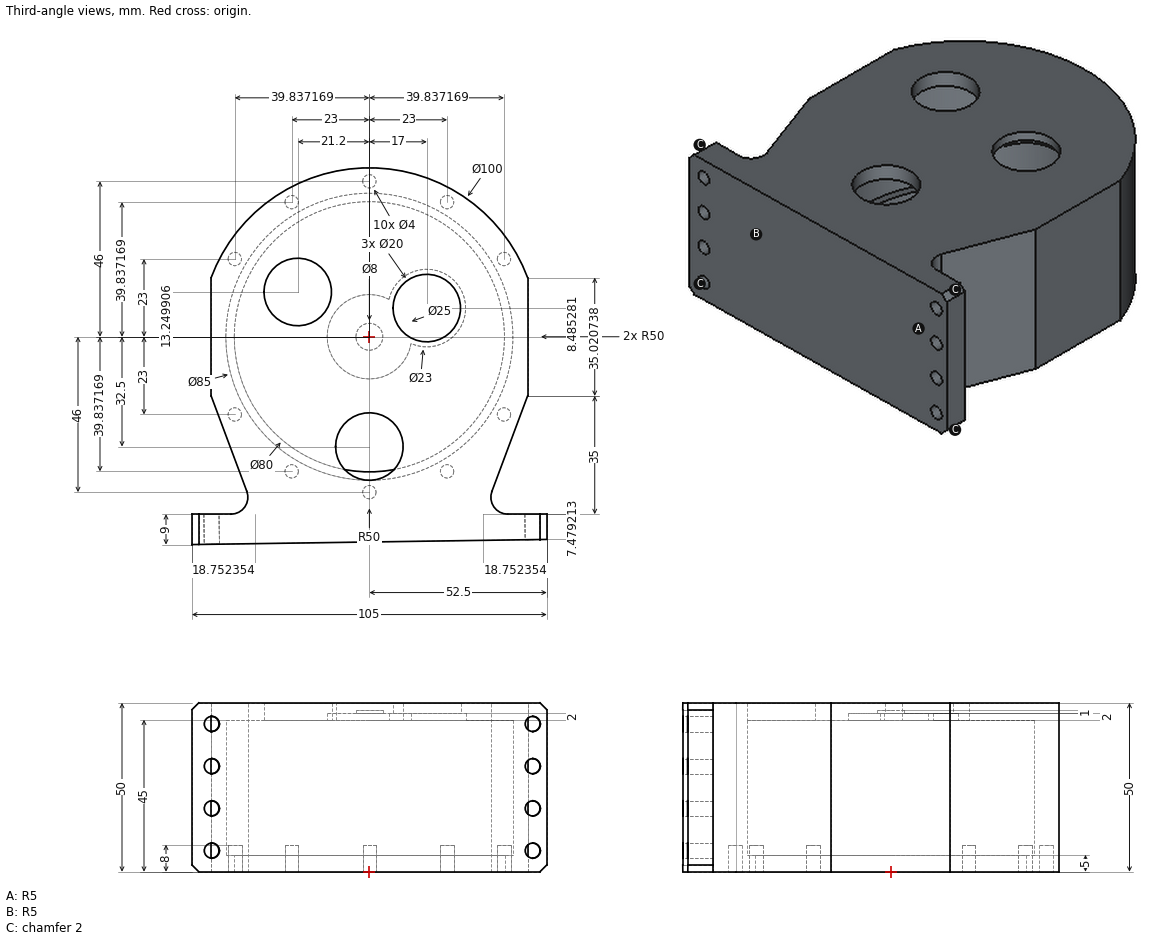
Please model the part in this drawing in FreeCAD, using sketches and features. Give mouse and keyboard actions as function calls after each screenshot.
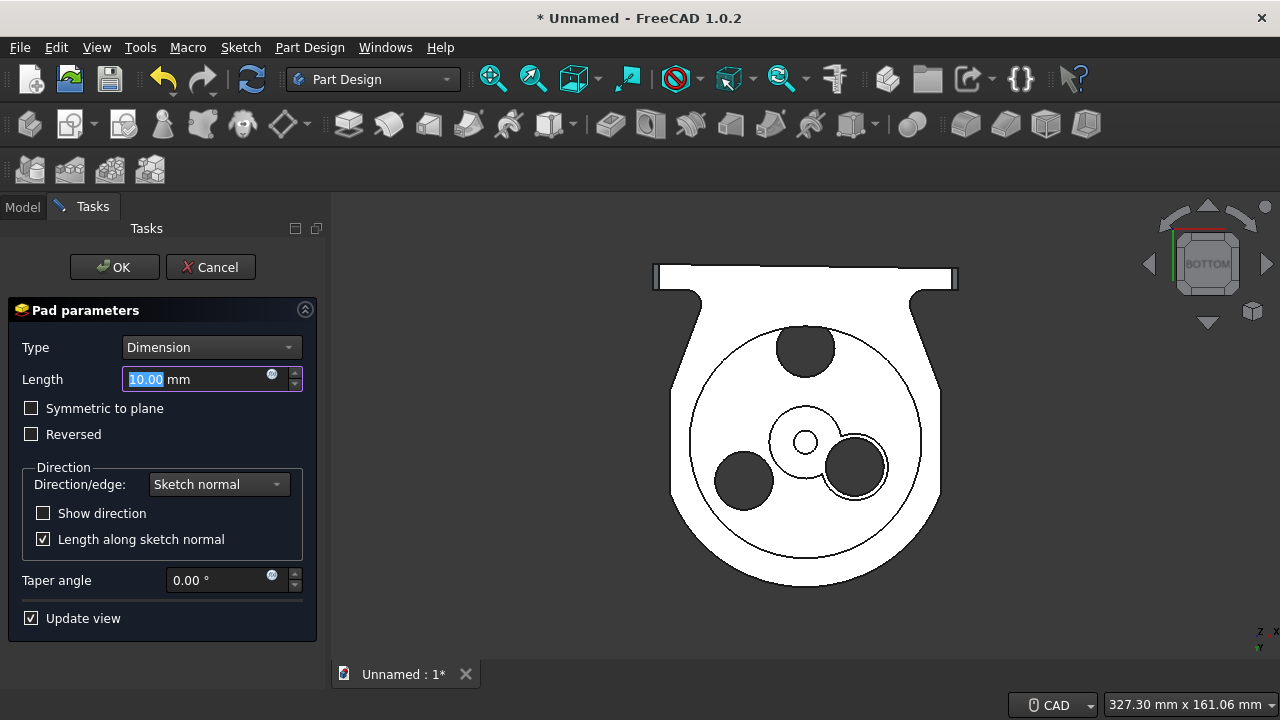
text(5)
key(Tab)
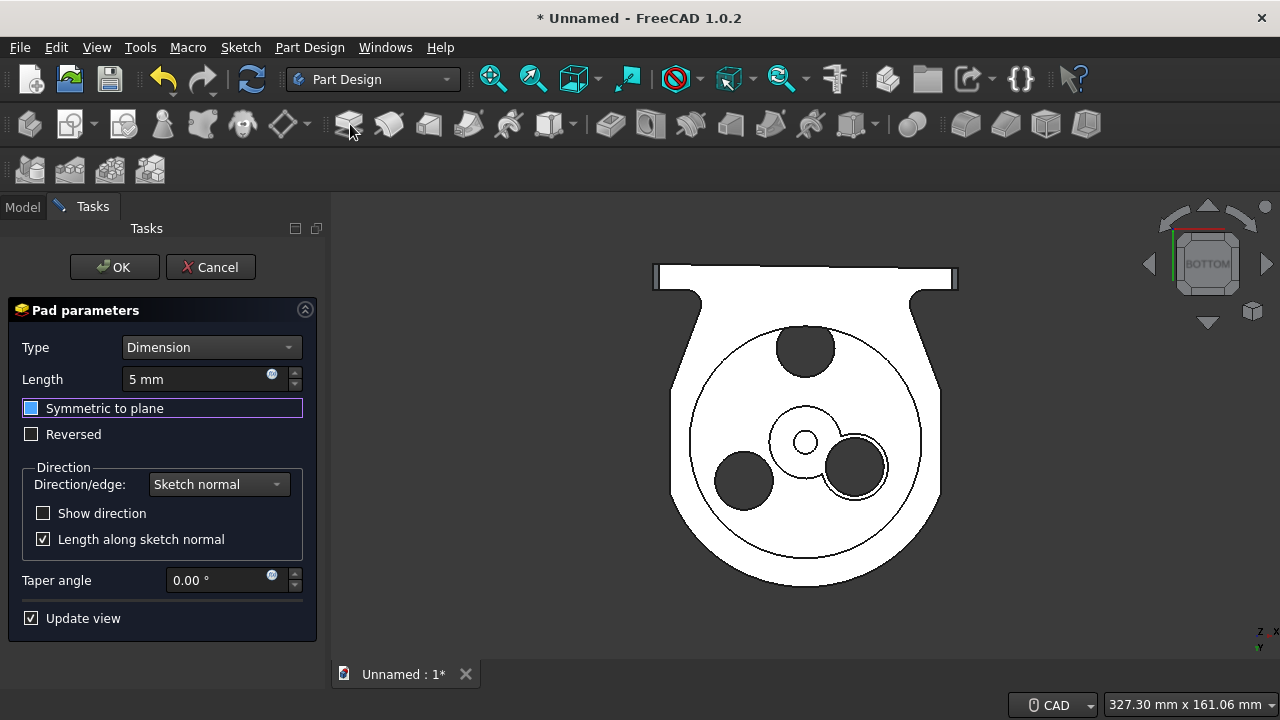
click(115, 267)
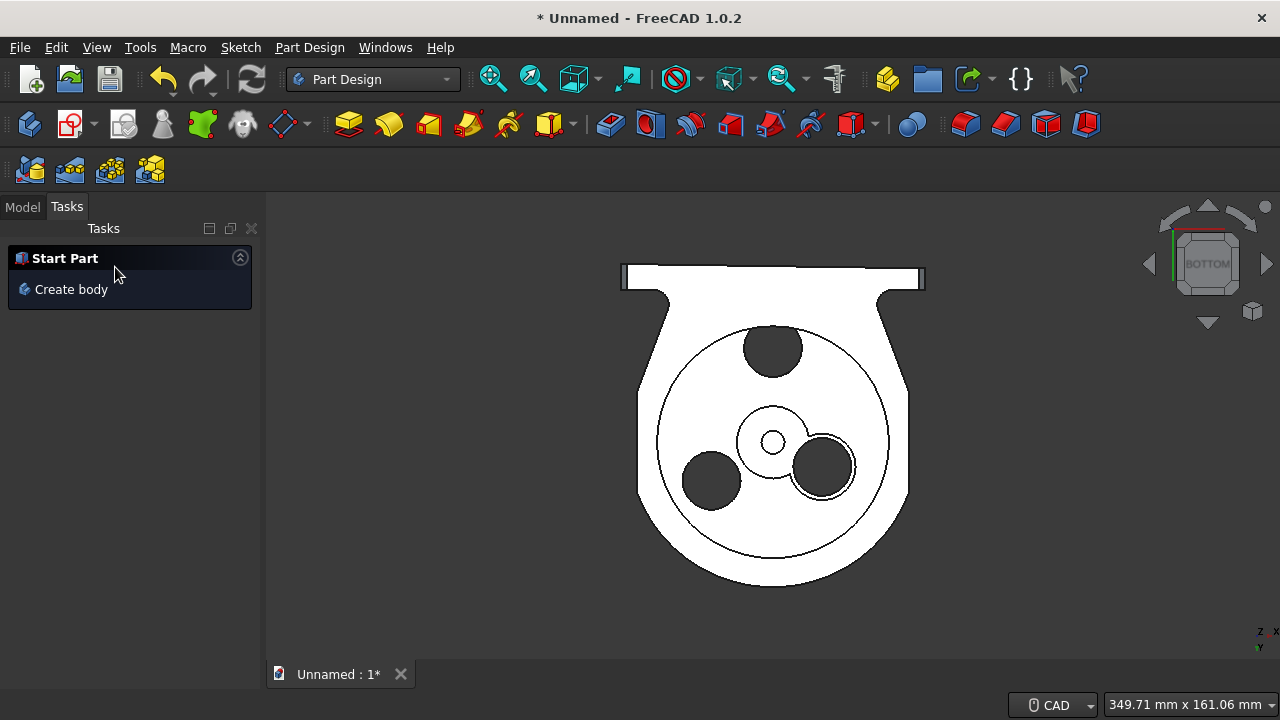
click(689, 286)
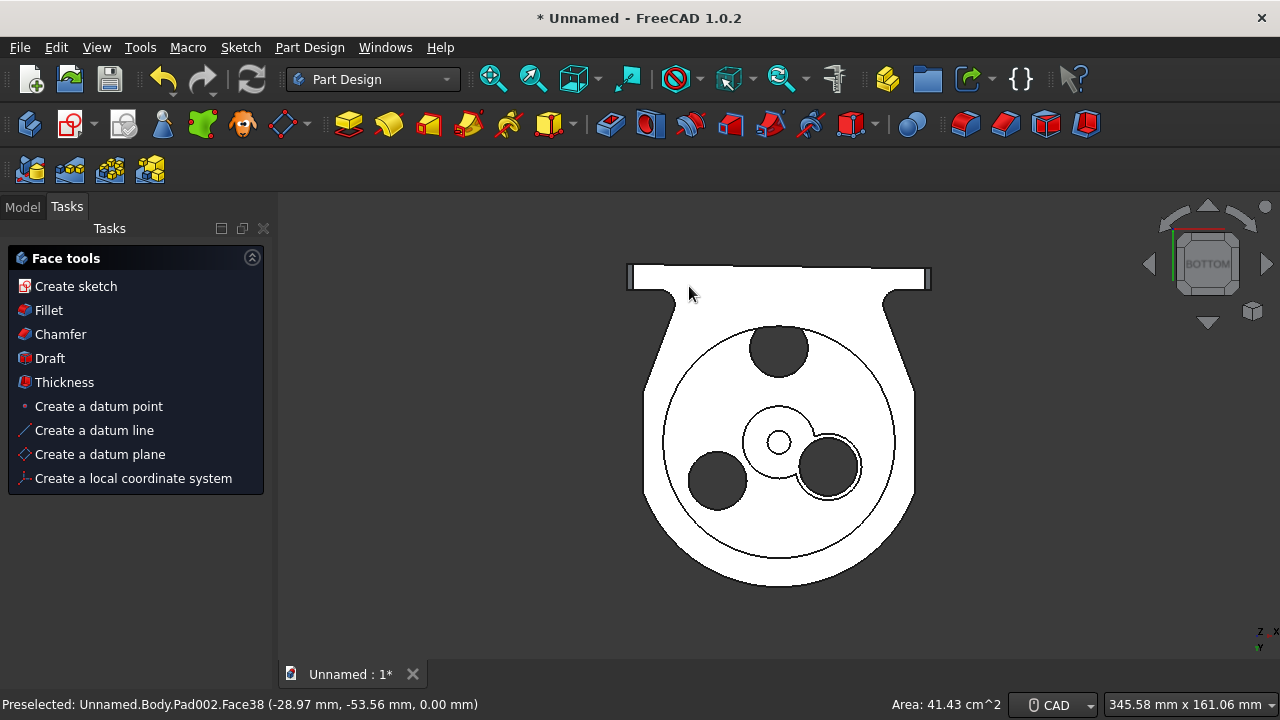
click(70, 124)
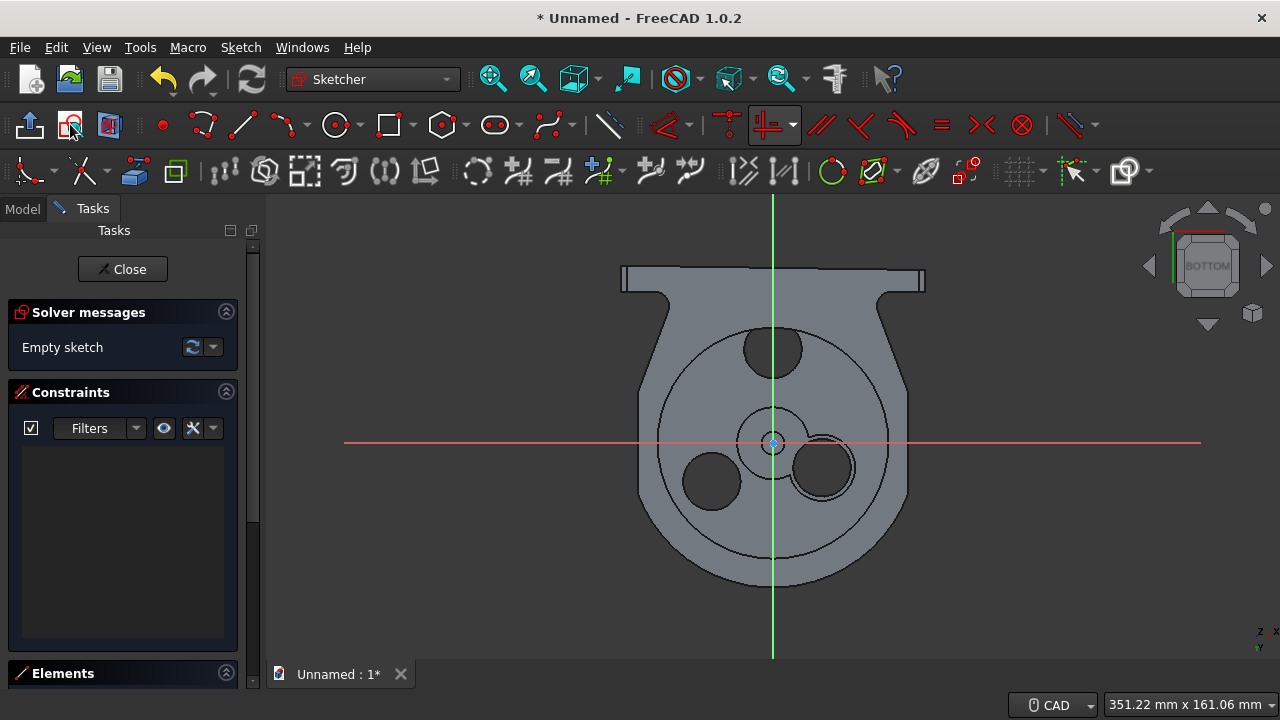
click(336, 126)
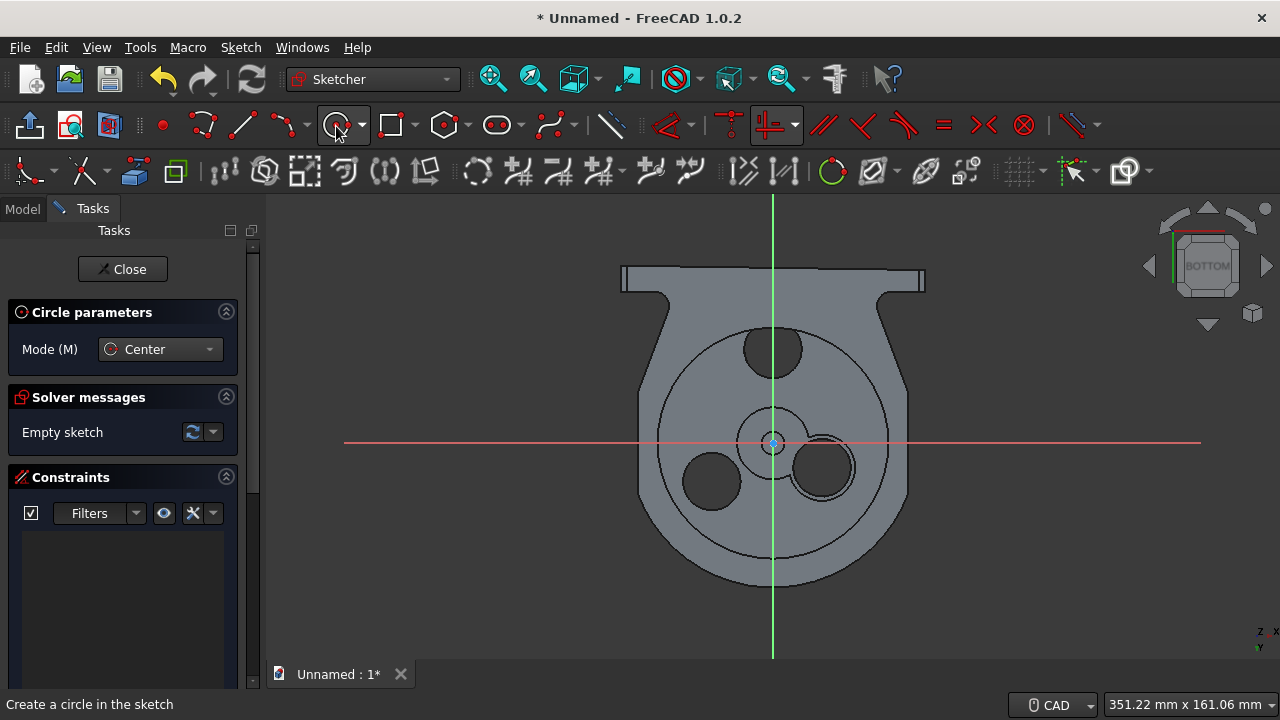
scroll(773, 576, up, 7)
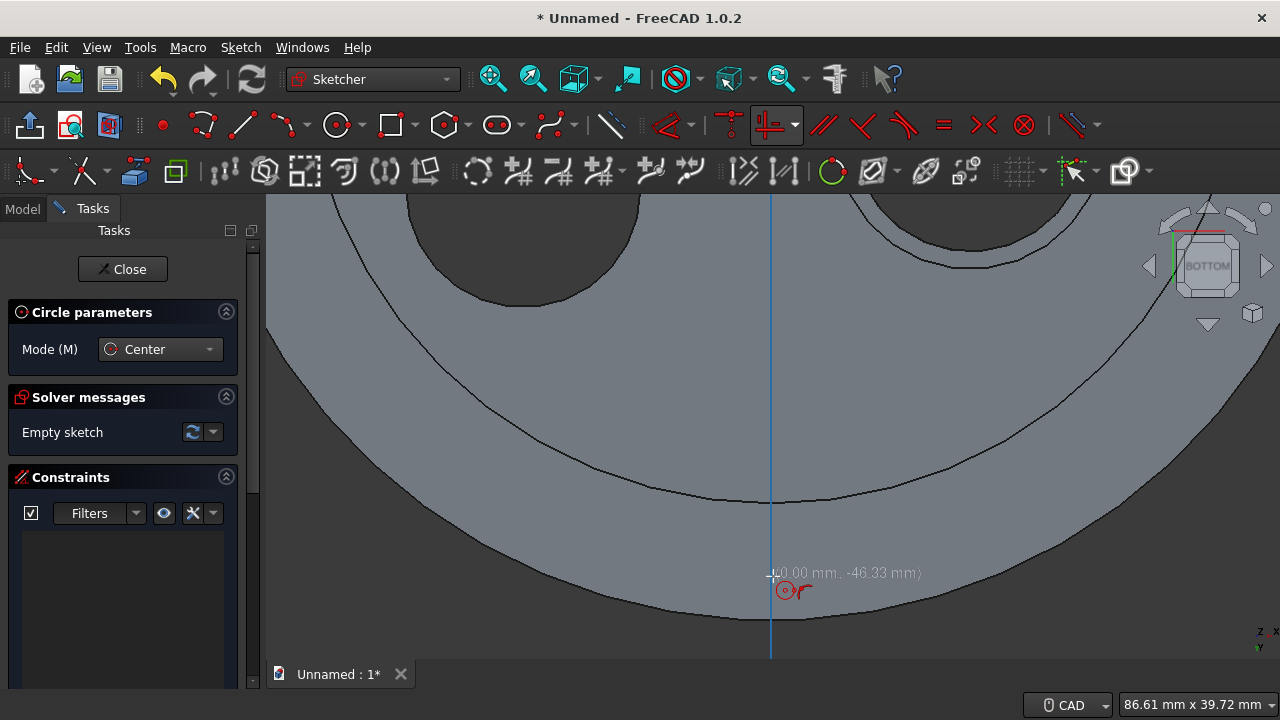
scroll(683, 555, down, 7)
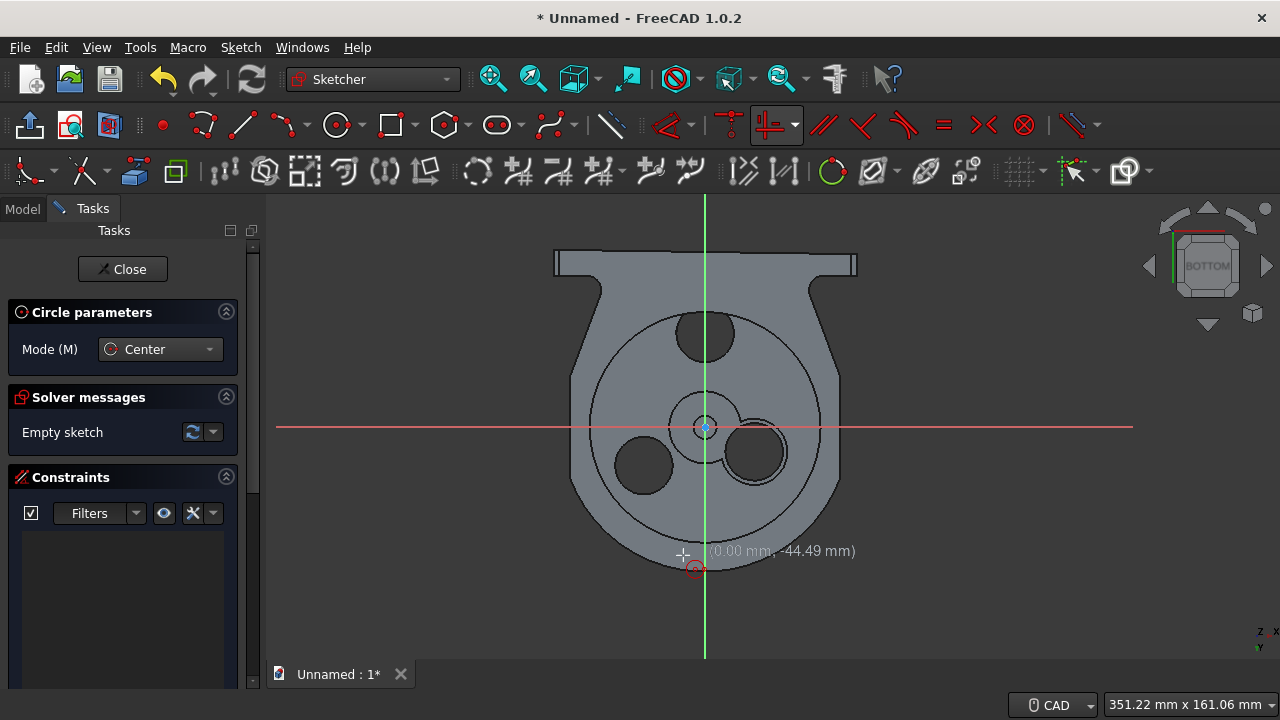
click(705, 560)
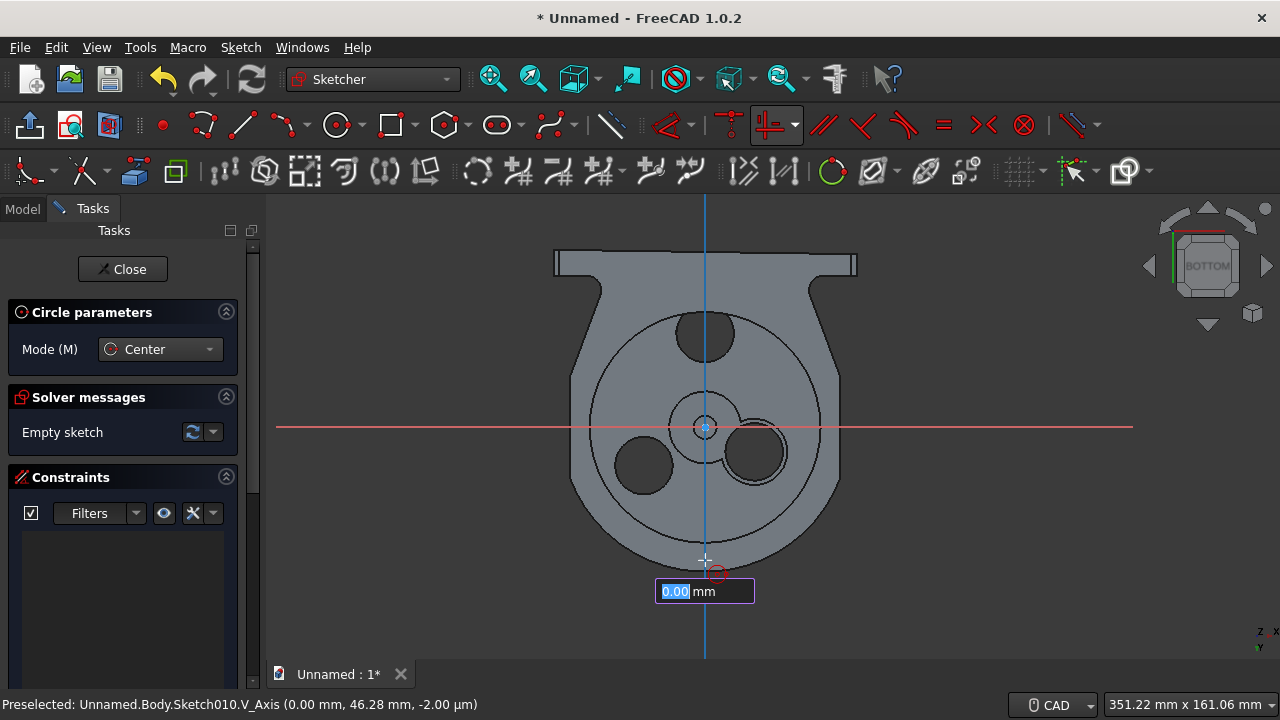
scroll(711, 558, up, 6)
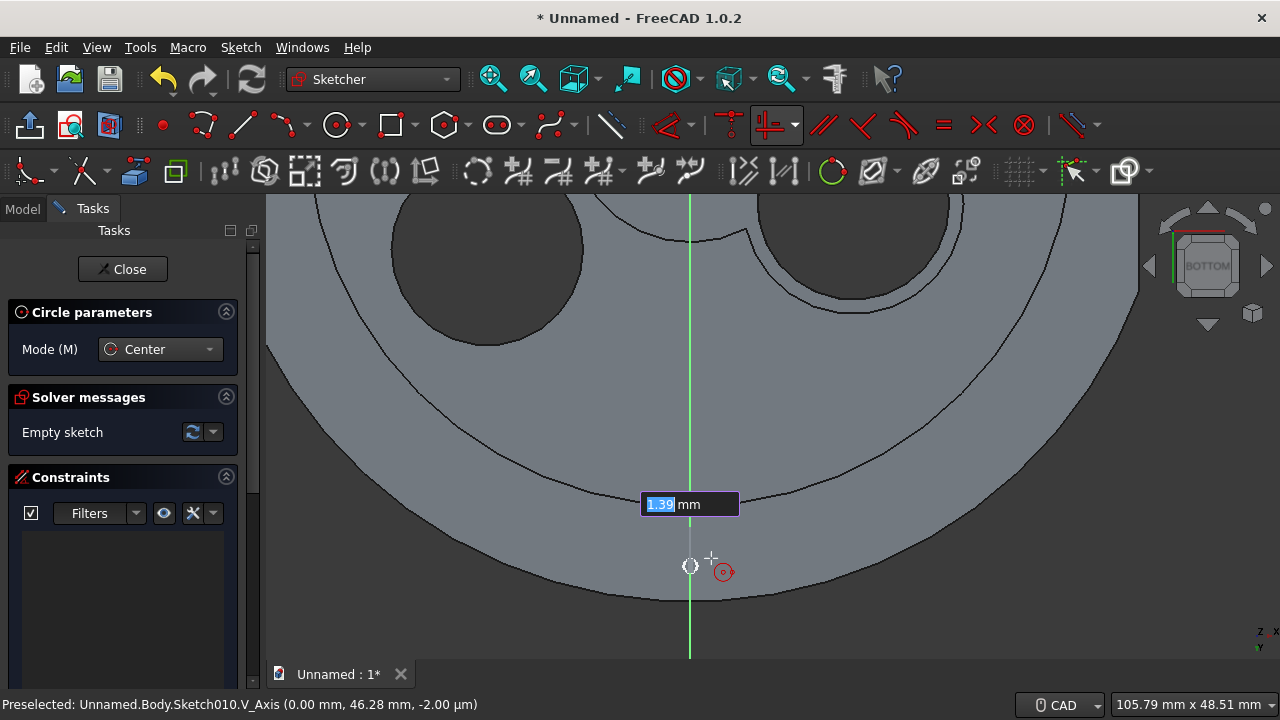
click(708, 557)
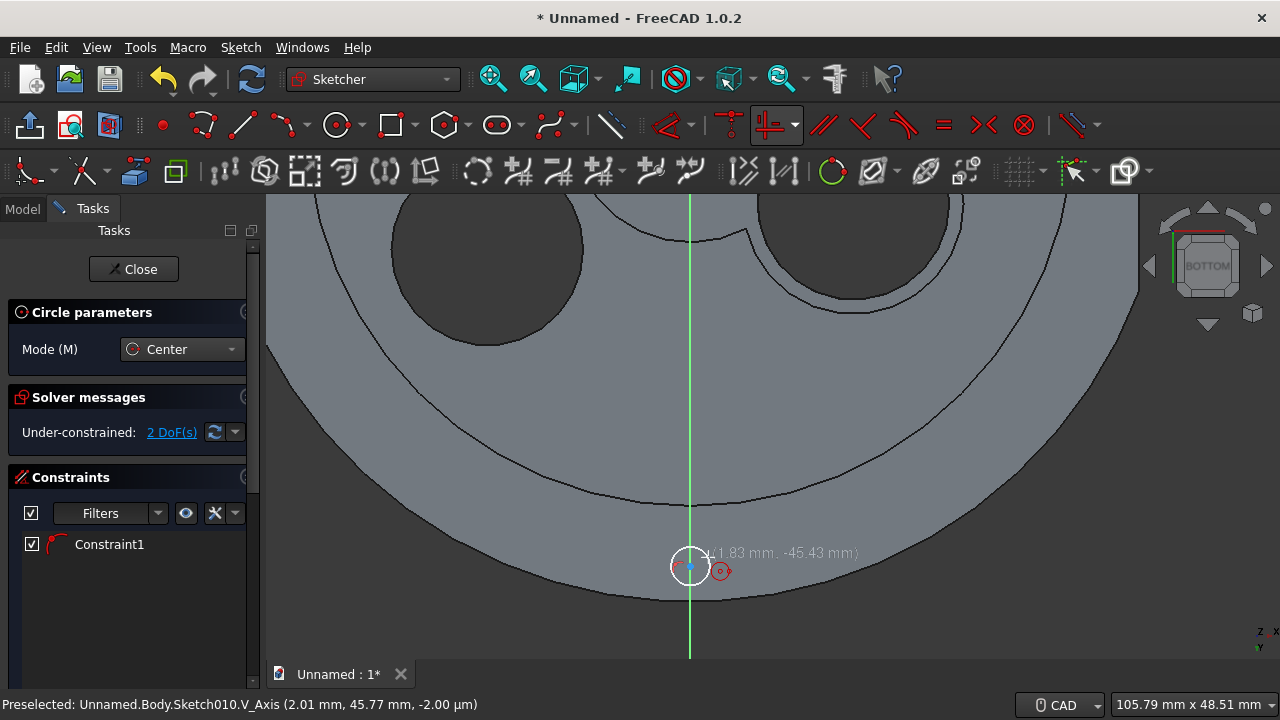
click(470, 504)
click(484, 491)